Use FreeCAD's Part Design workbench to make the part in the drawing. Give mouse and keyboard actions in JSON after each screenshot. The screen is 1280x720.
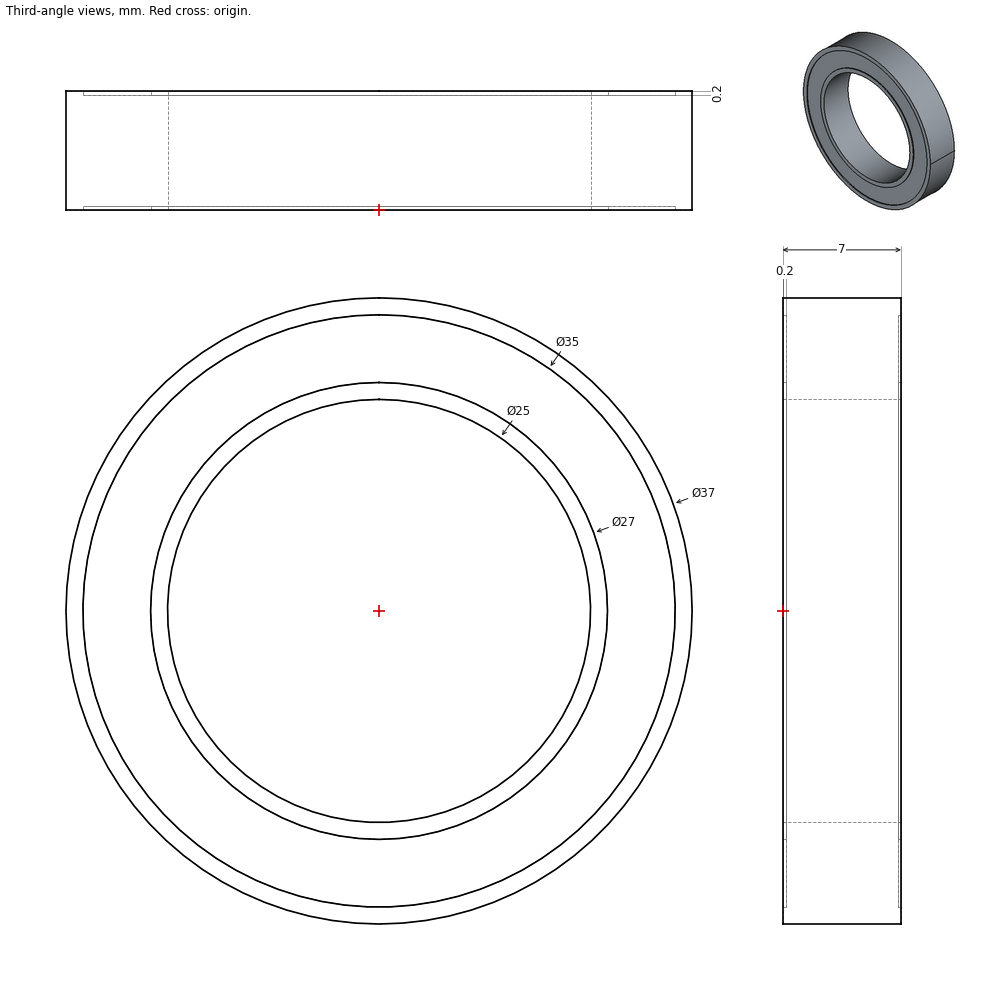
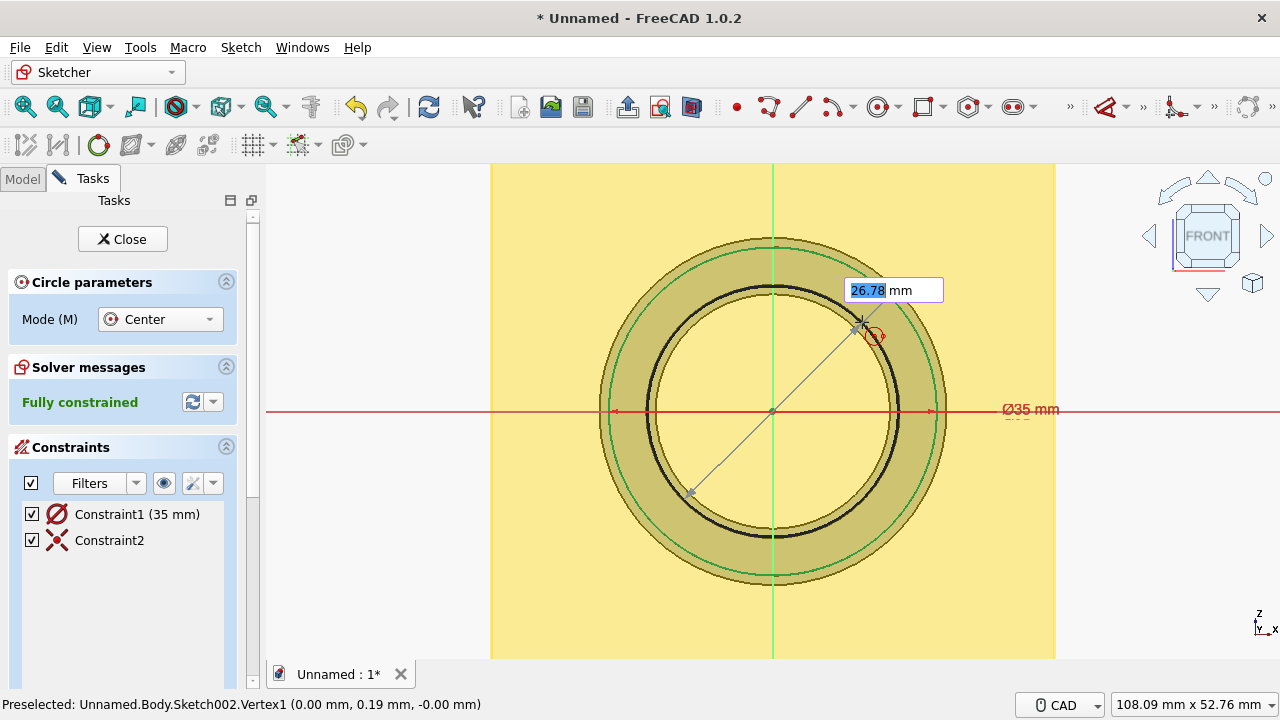
{"action": "type", "text": "27"}
{"action": "key", "text": "Return"}
{"action": "key", "text": "Escape"}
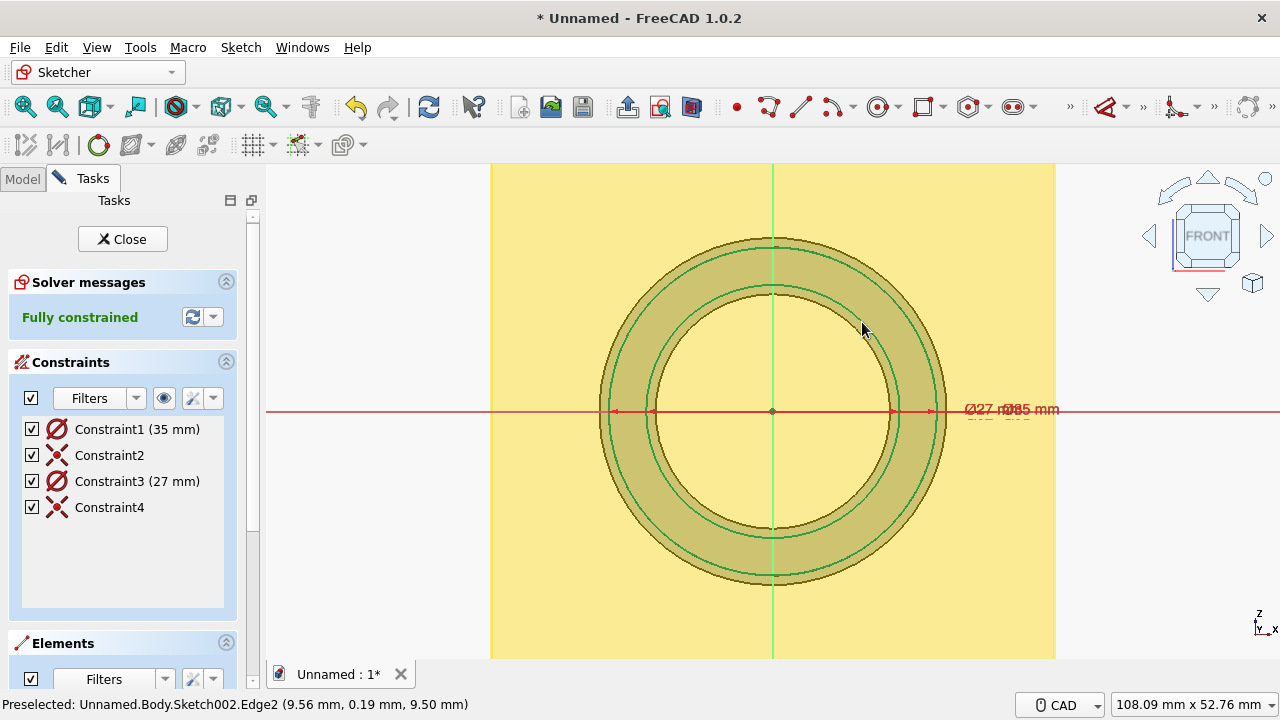
{"action": "left_click", "coordinate": [123, 239]}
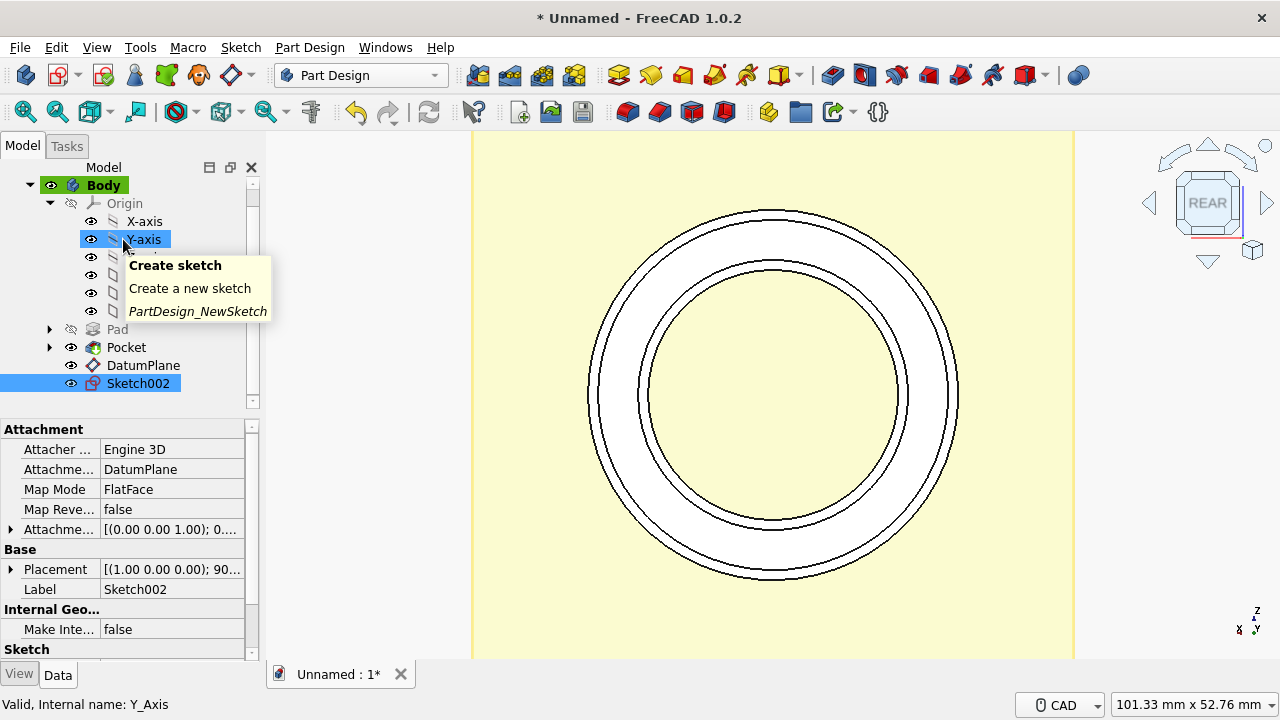
{"action": "left_click", "coordinate": [834, 76]}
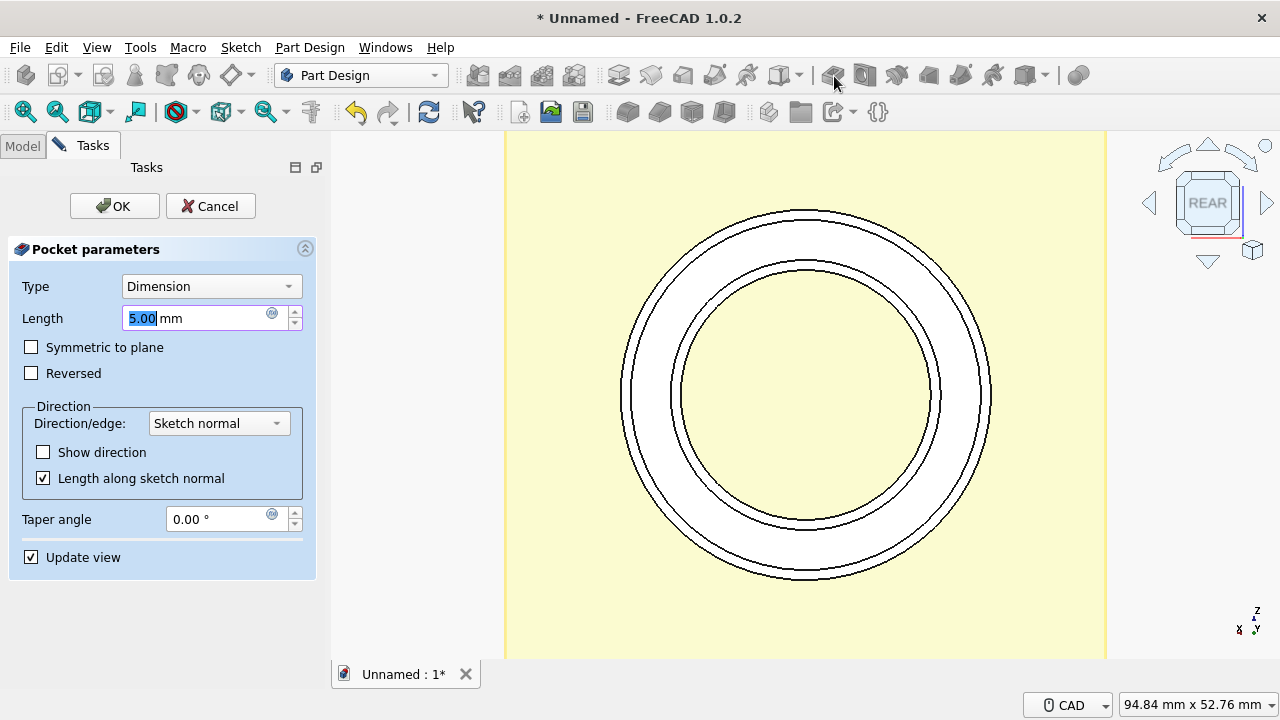
{"action": "type", "text": "0.2"}
{"action": "key", "text": "Tab"}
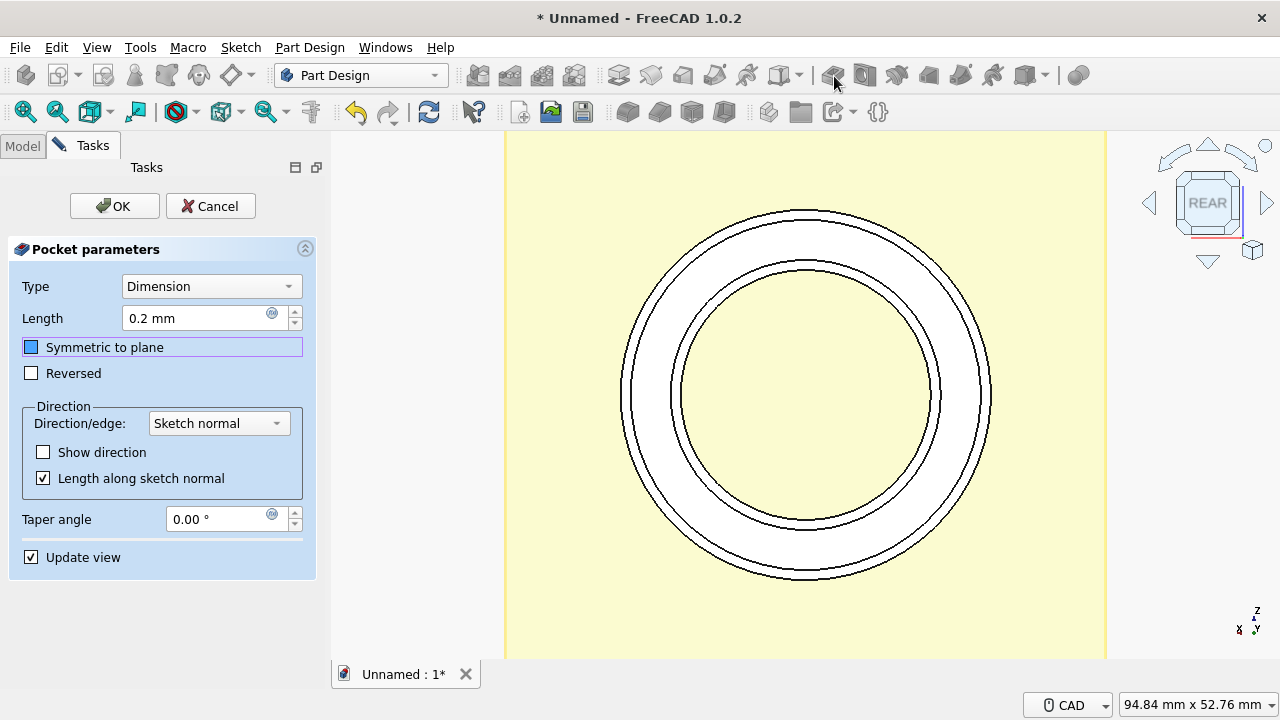
{"action": "left_click", "coordinate": [30, 373]}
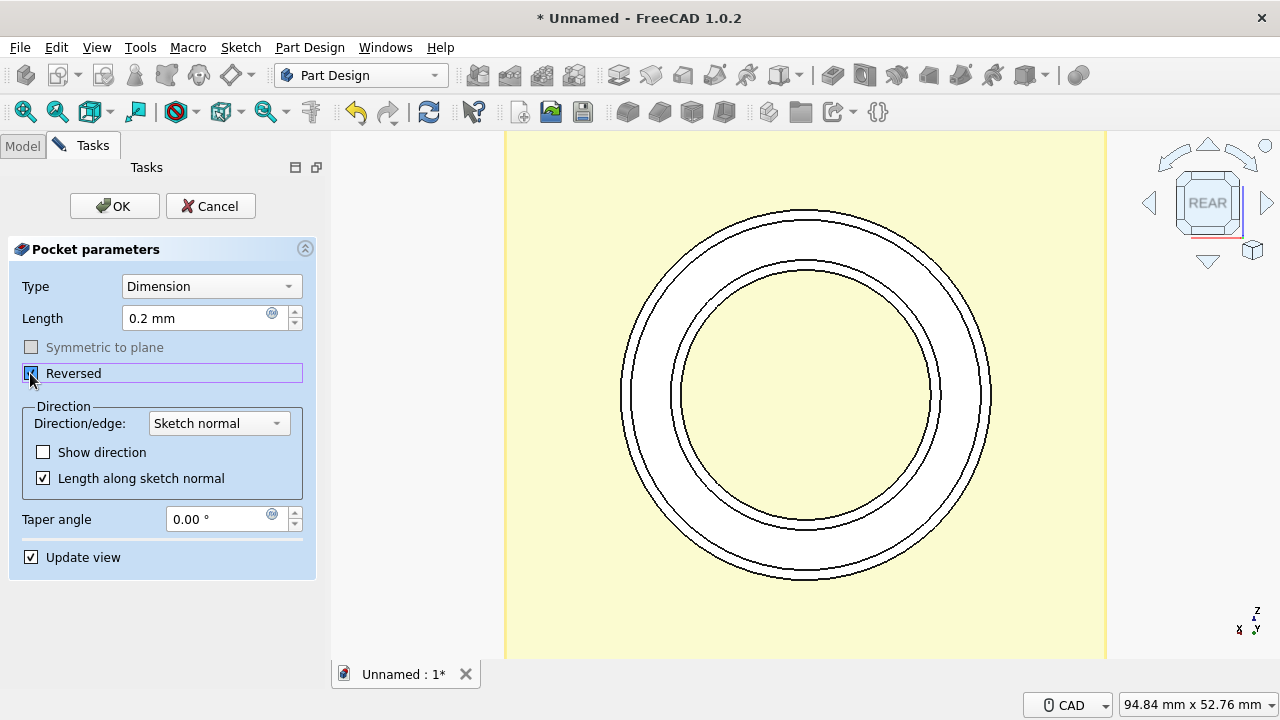
{"action": "left_click", "coordinate": [115, 206]}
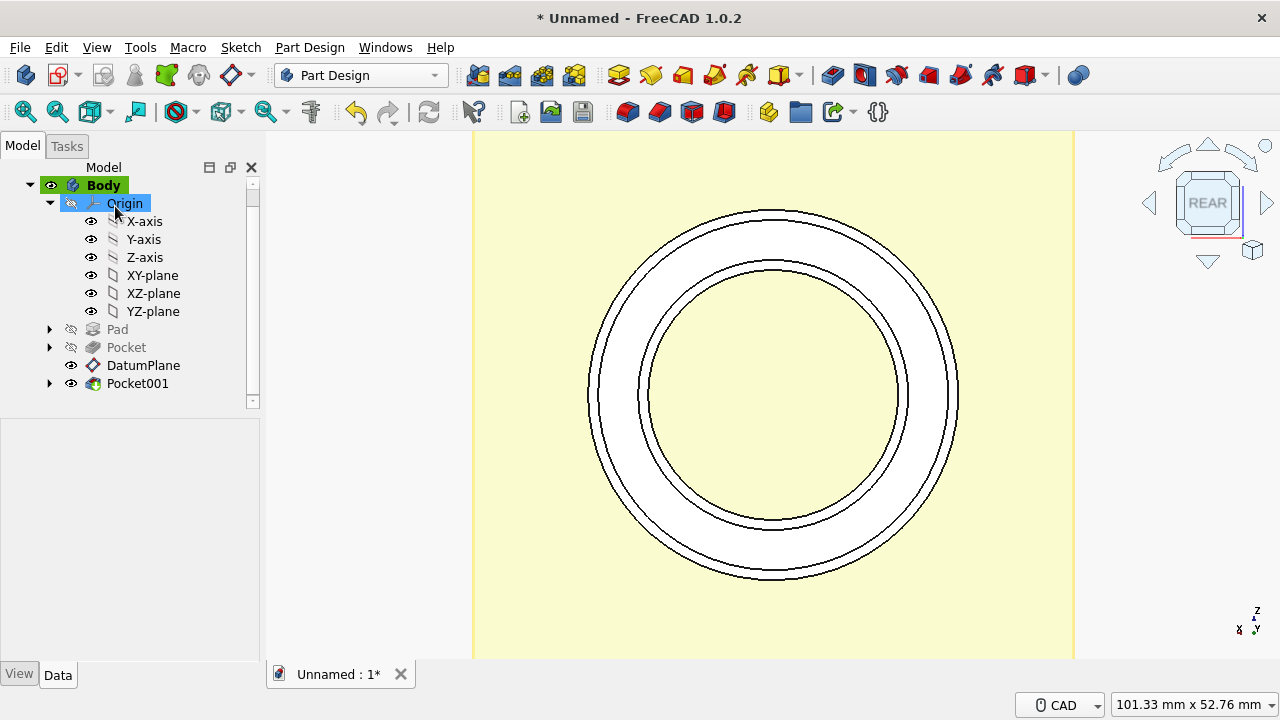
{"action": "left_click", "coordinate": [116, 365]}
{"action": "key", "text": "space"}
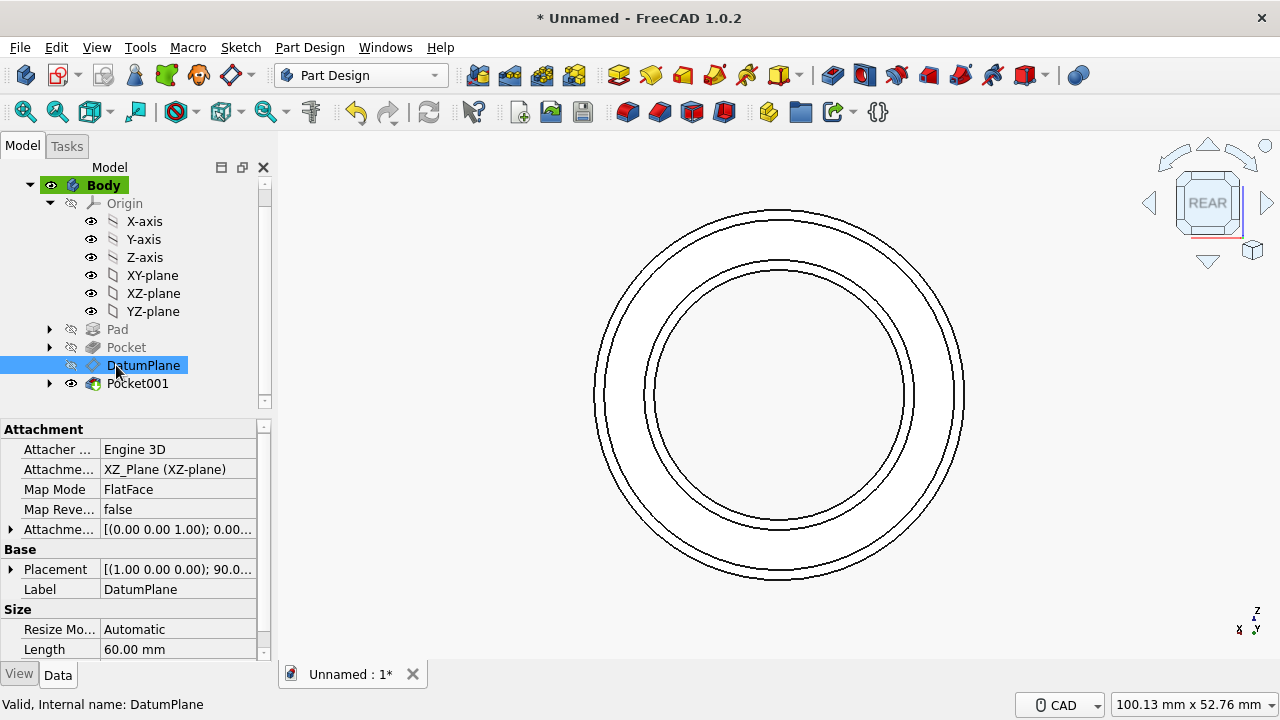
{"action": "key", "text": "0"}